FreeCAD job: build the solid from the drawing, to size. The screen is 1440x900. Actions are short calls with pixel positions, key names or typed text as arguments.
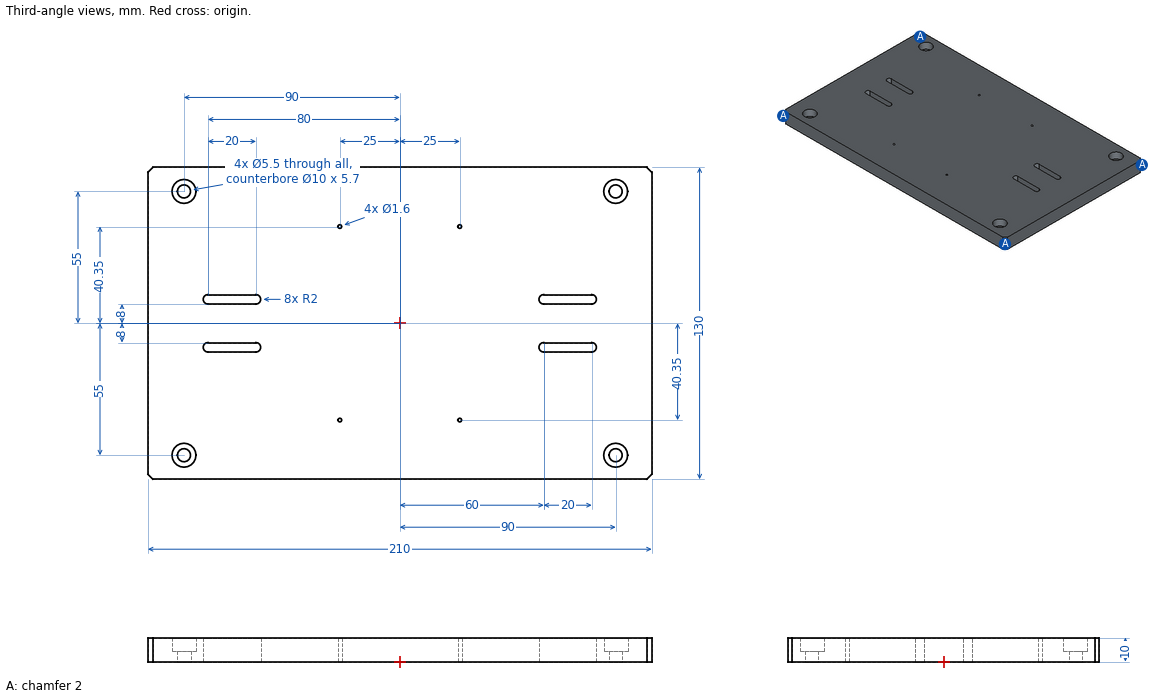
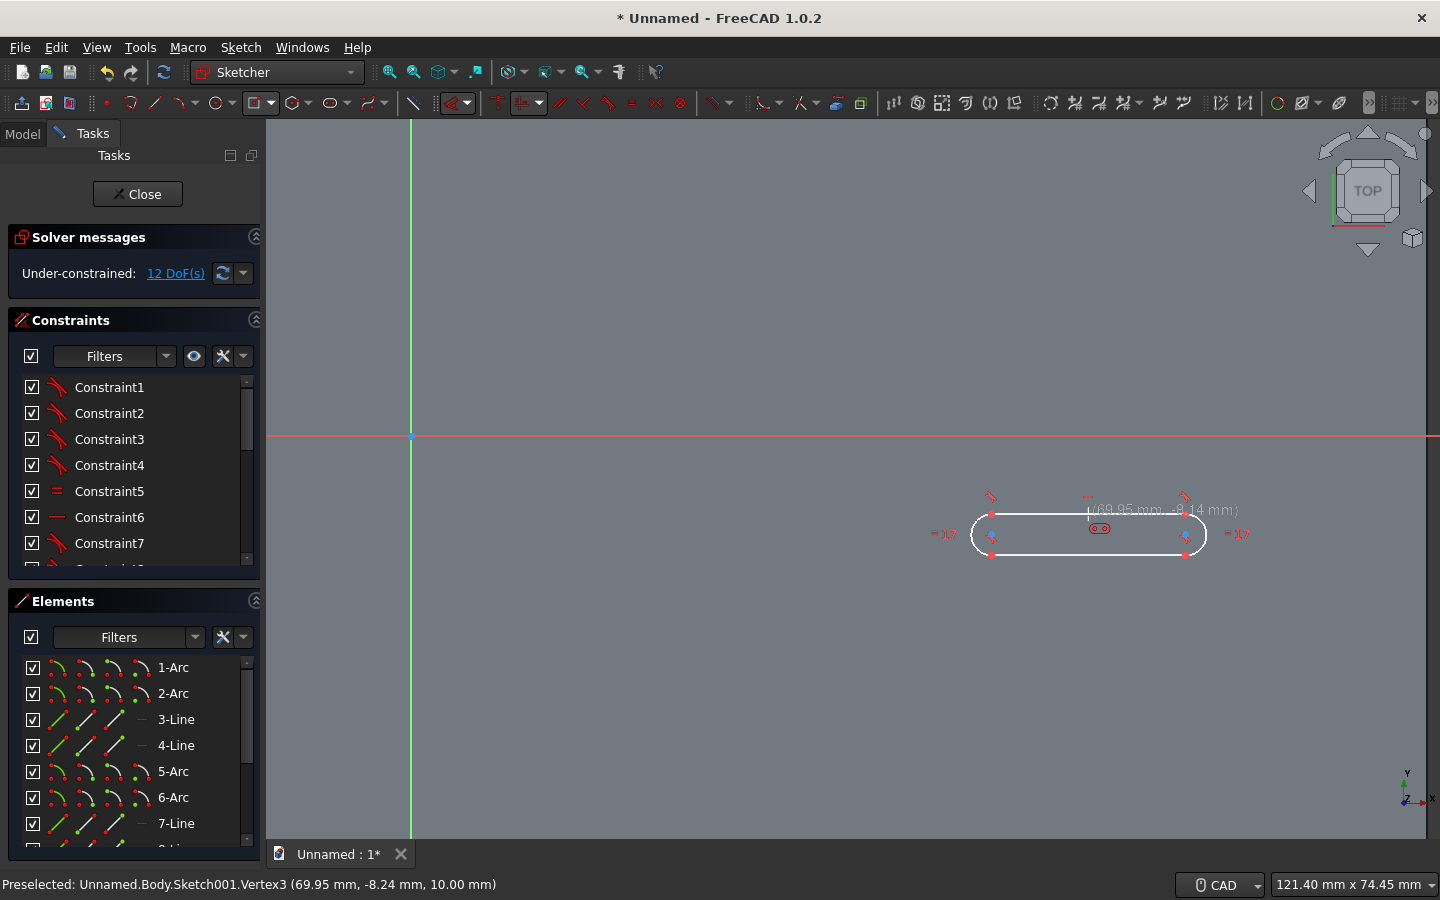
click(992, 340)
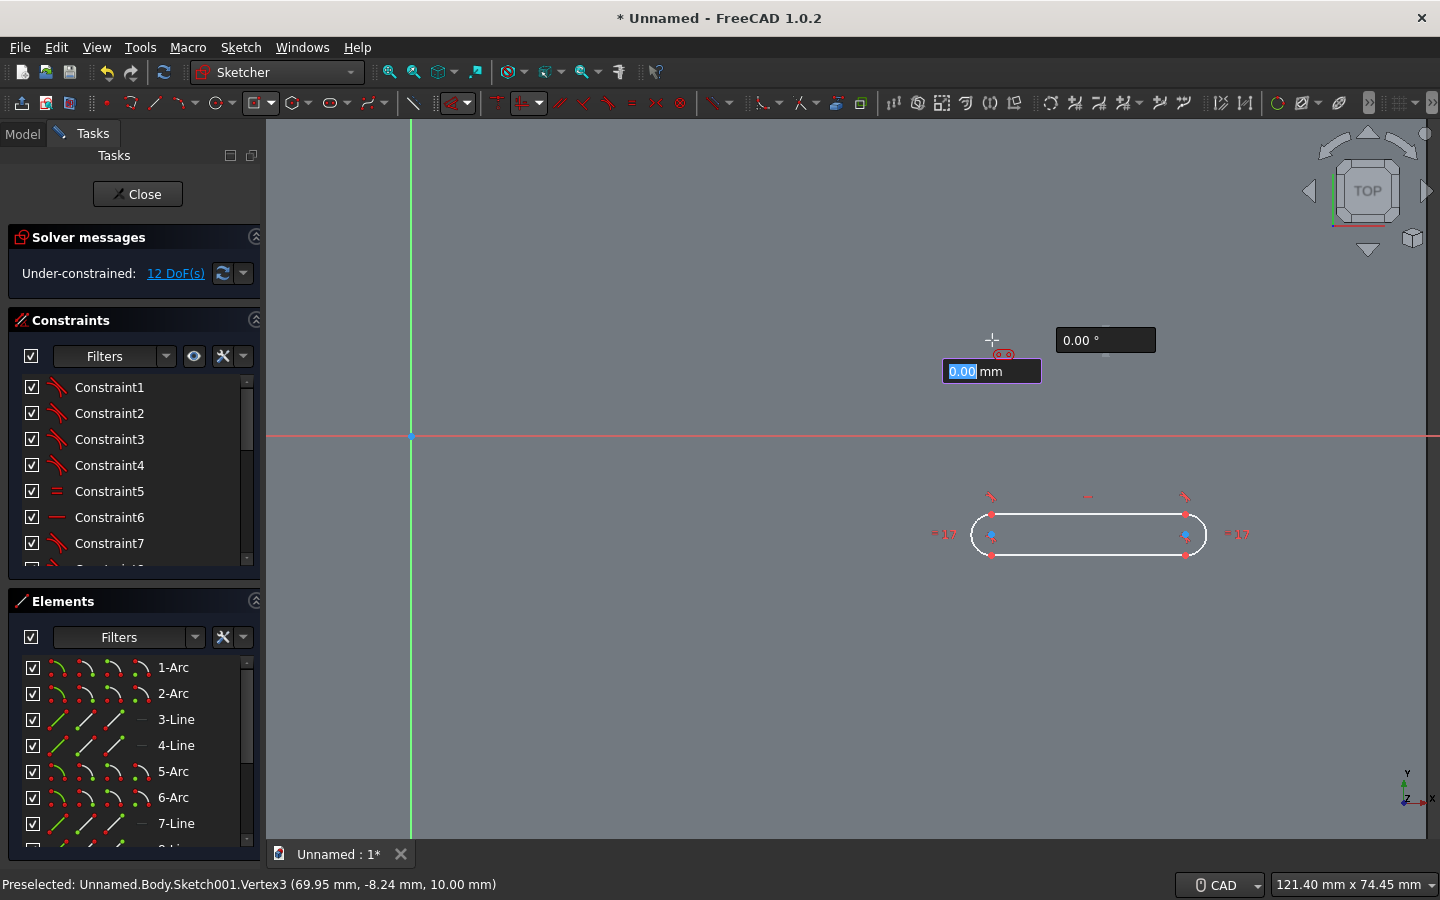
click(1185, 340)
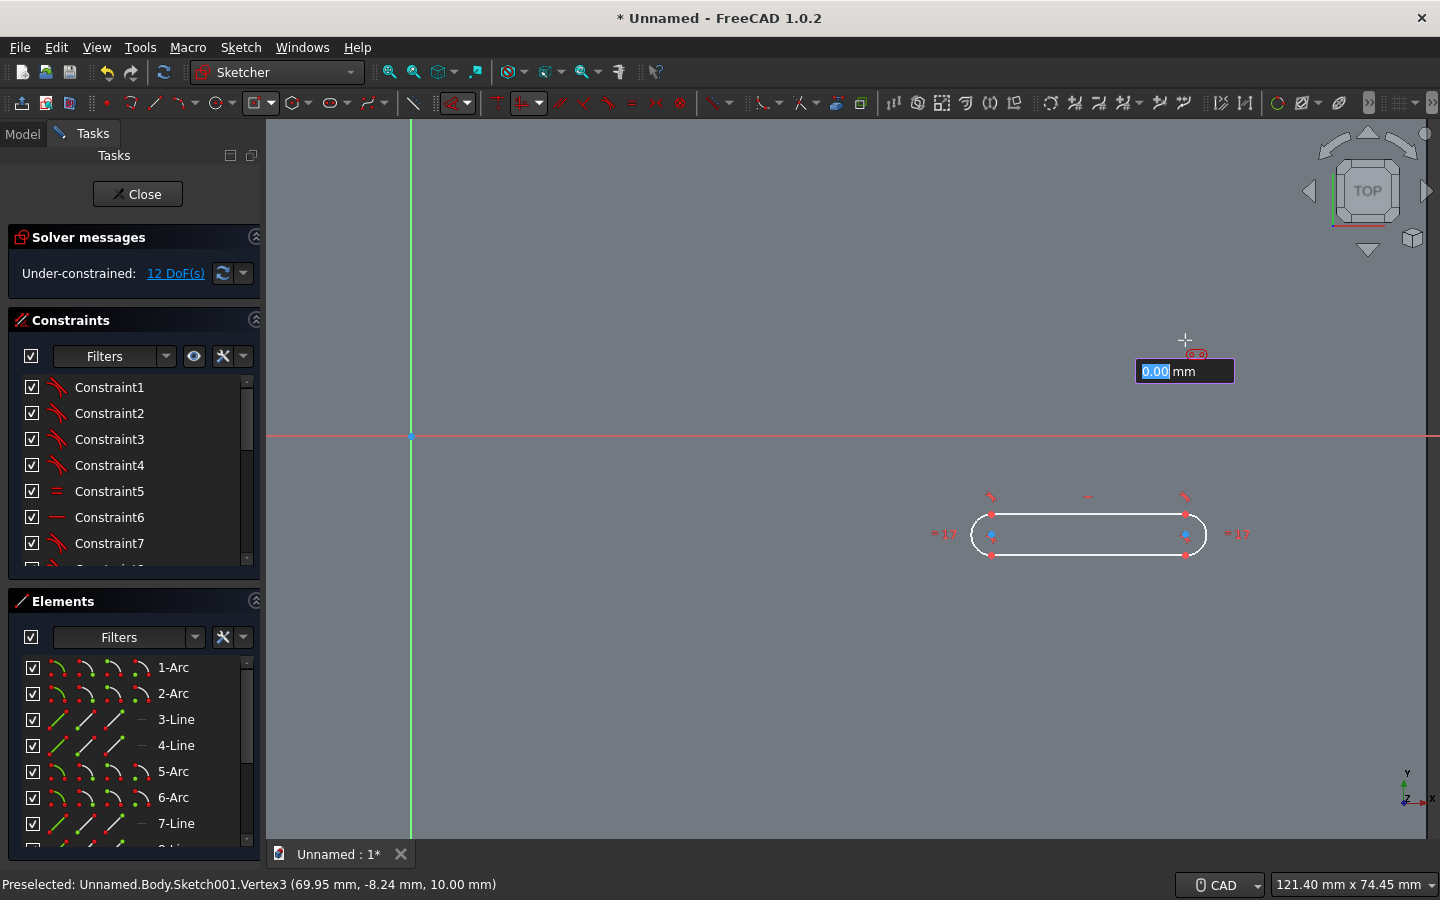
click(1088, 320)
key(Escape)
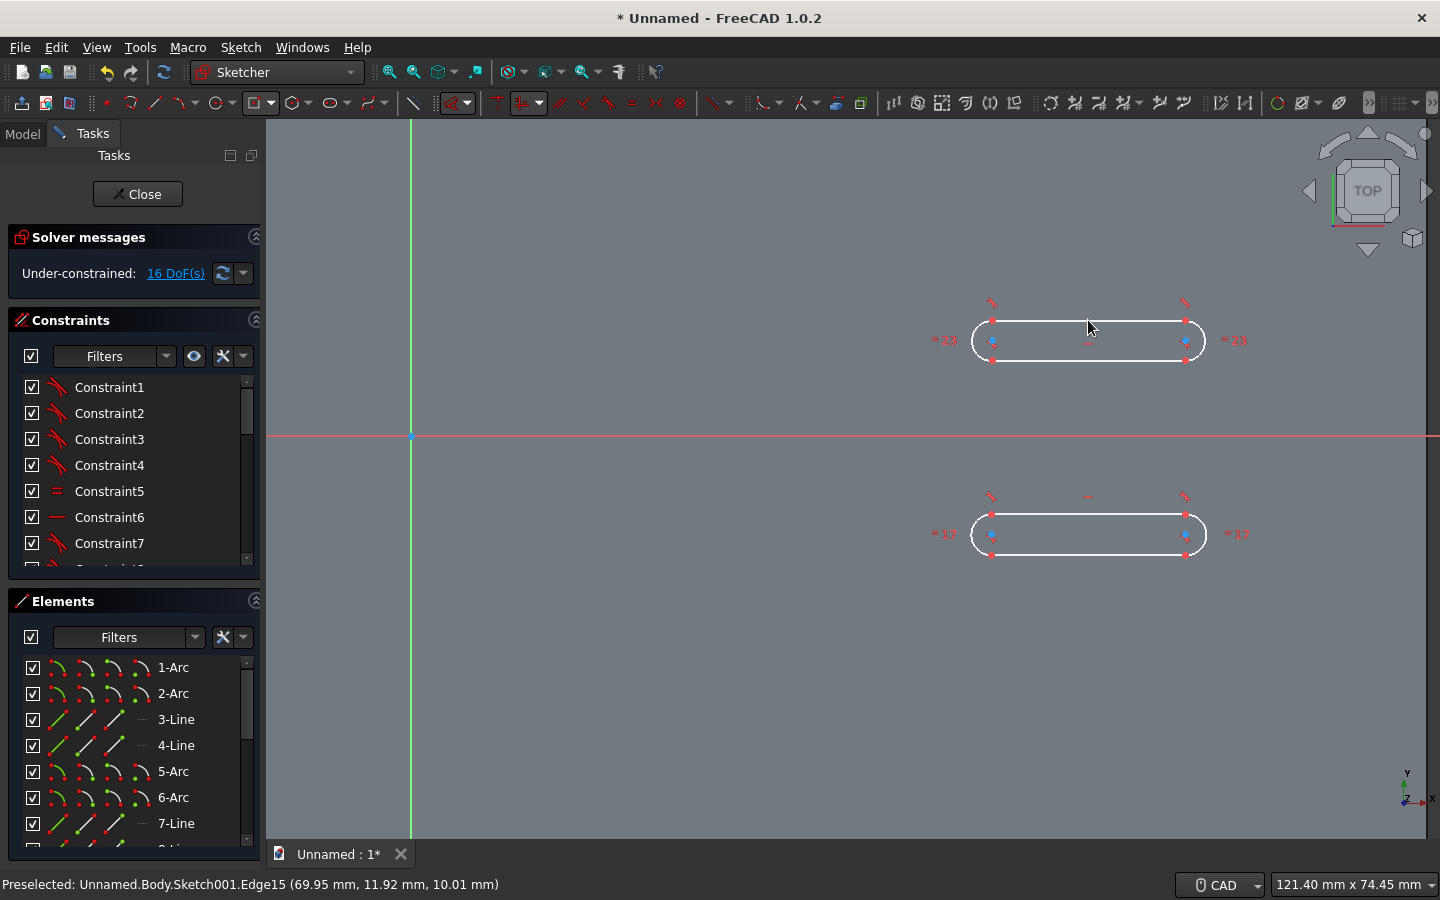
scroll(1089, 514, down, 4)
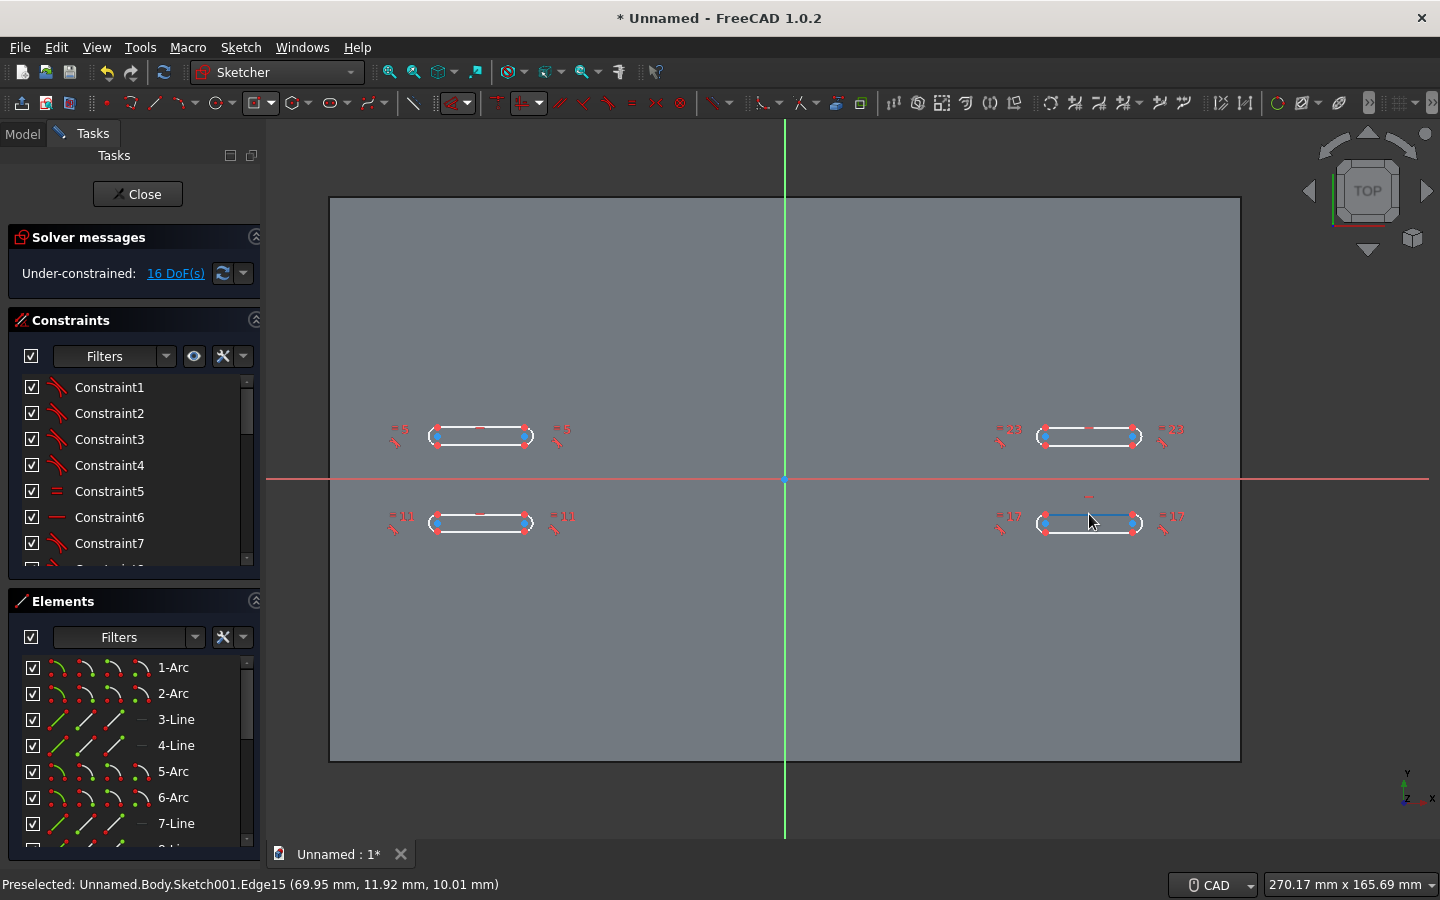
scroll(430, 431, up, 3)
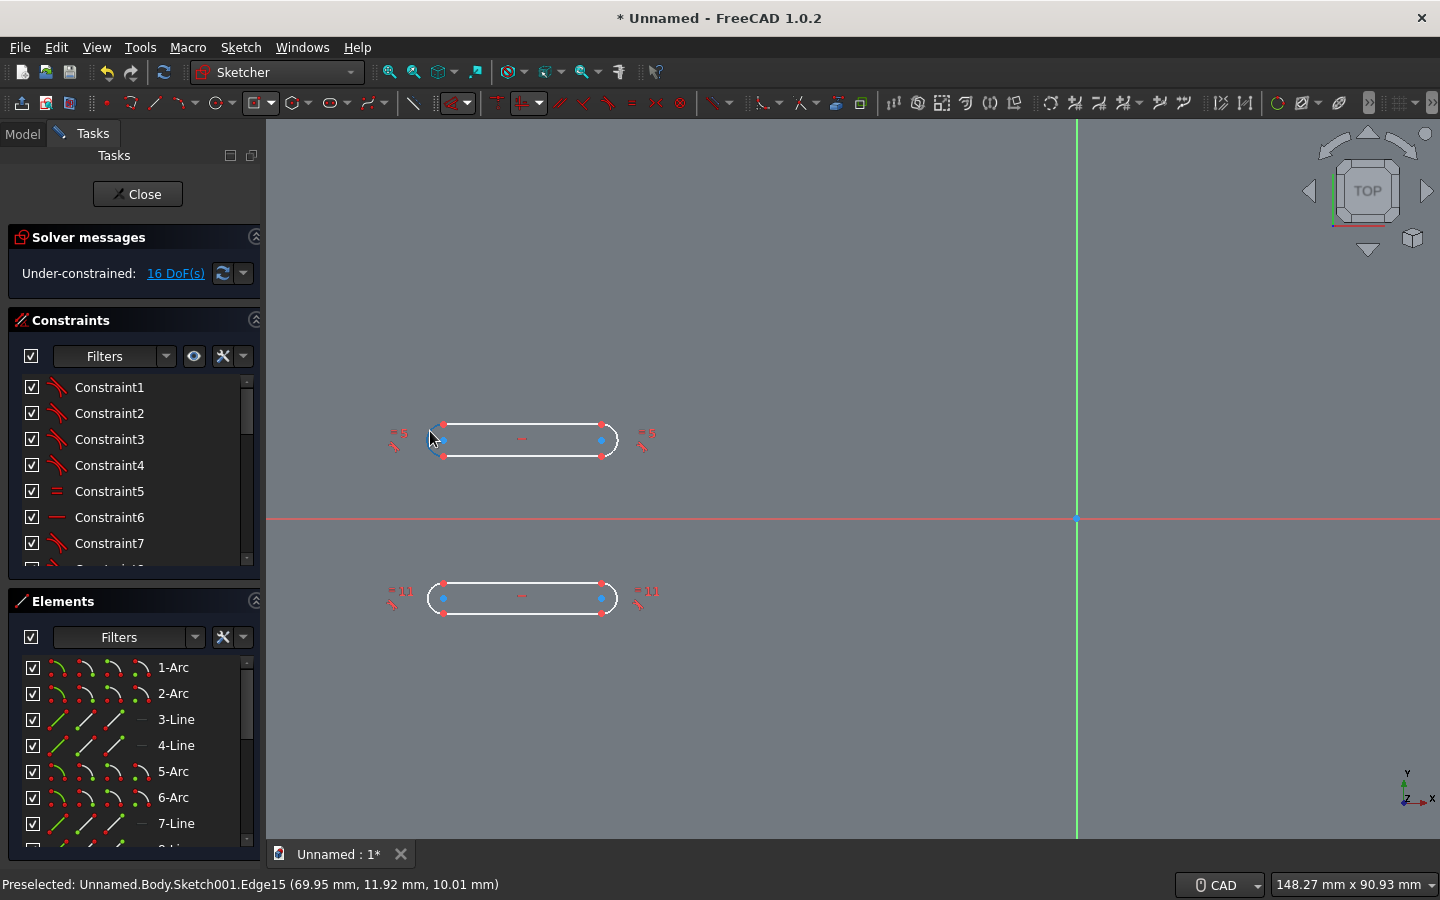
click(430, 431)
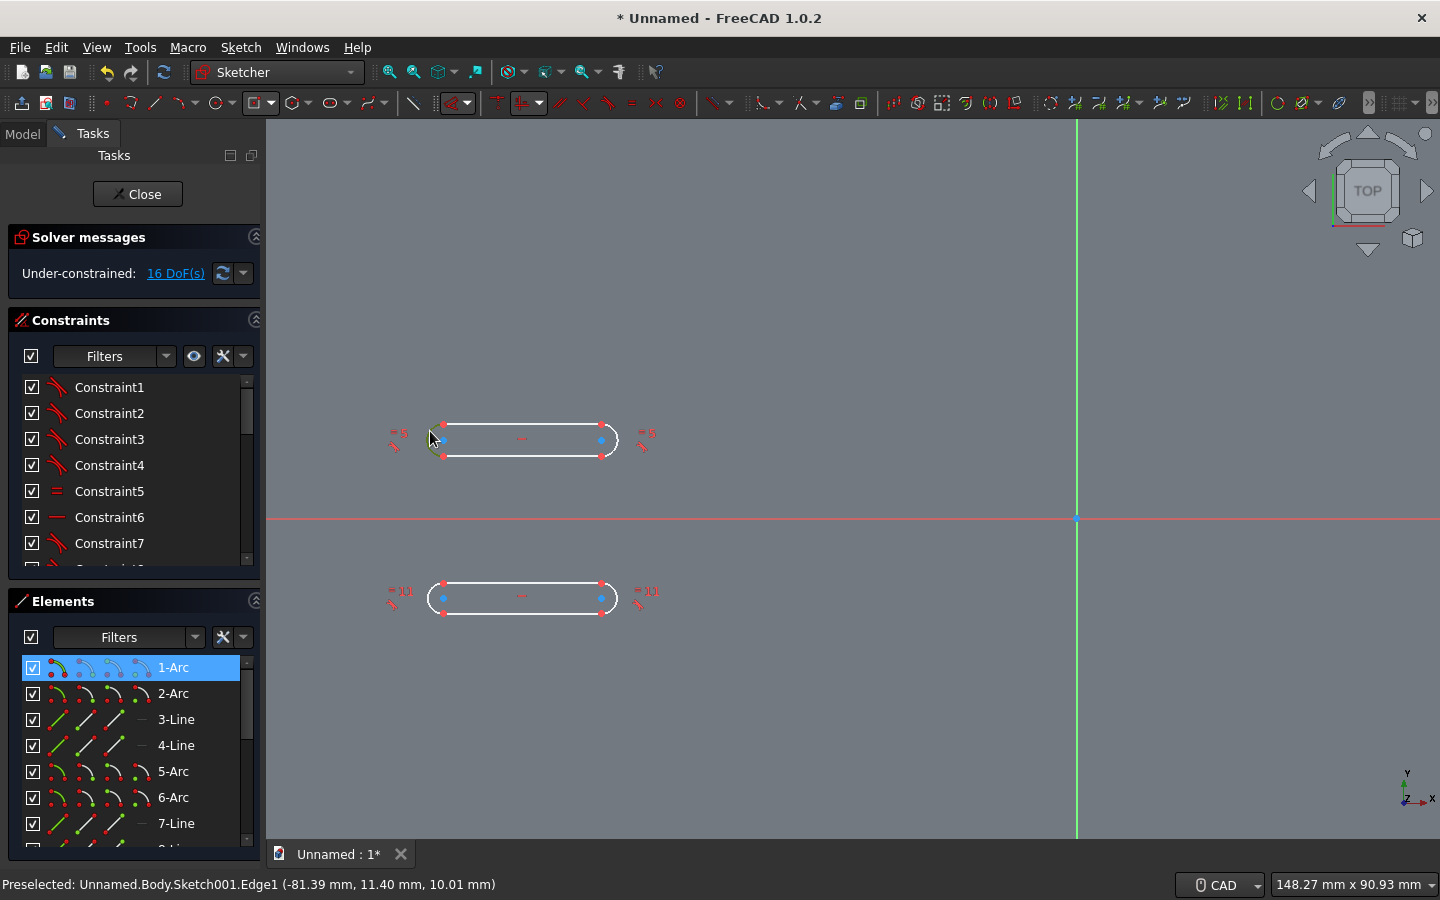
click(431, 589)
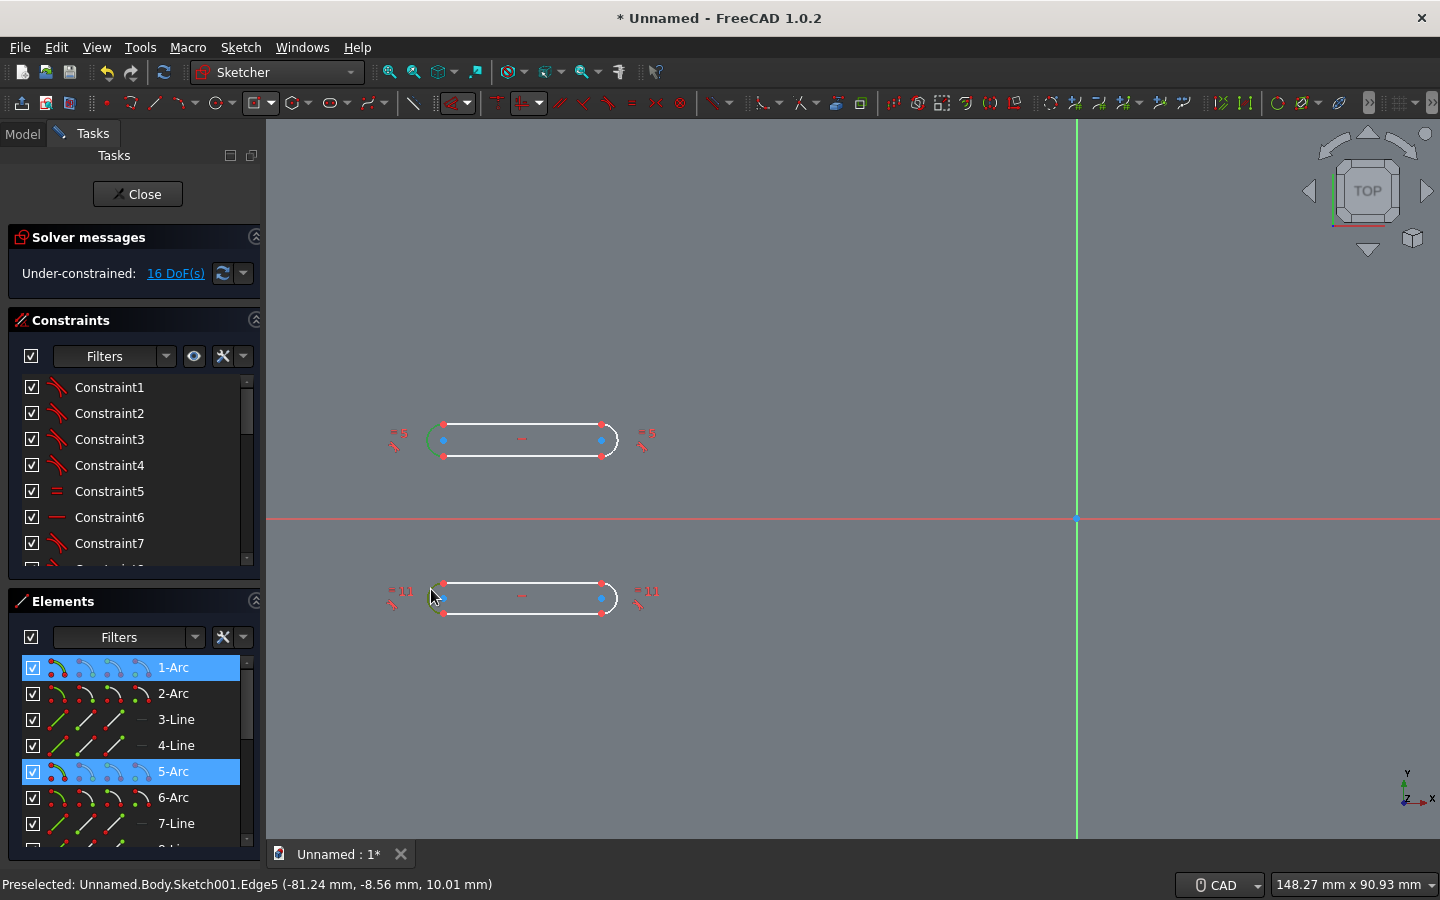
scroll(429, 431, down, 3)